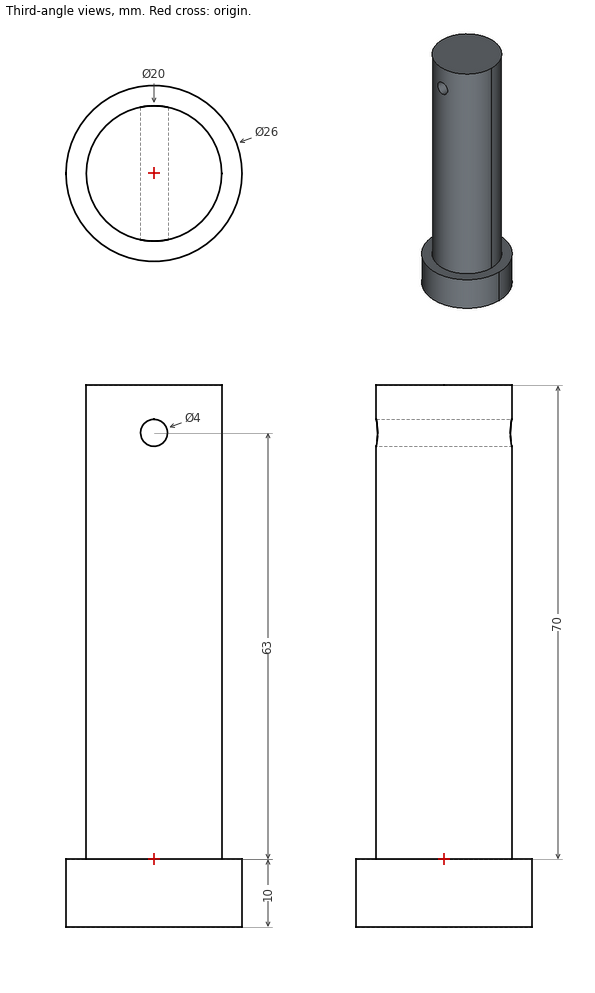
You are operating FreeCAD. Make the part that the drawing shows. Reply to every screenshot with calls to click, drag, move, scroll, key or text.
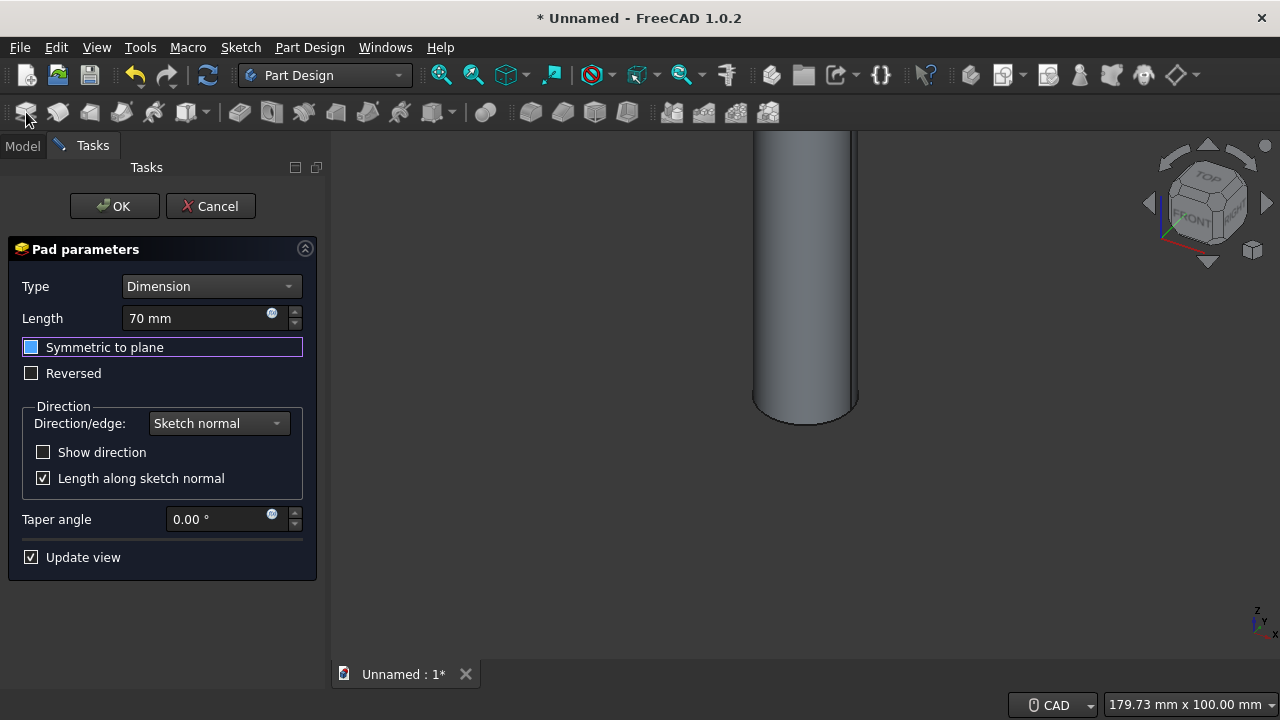
click(115, 206)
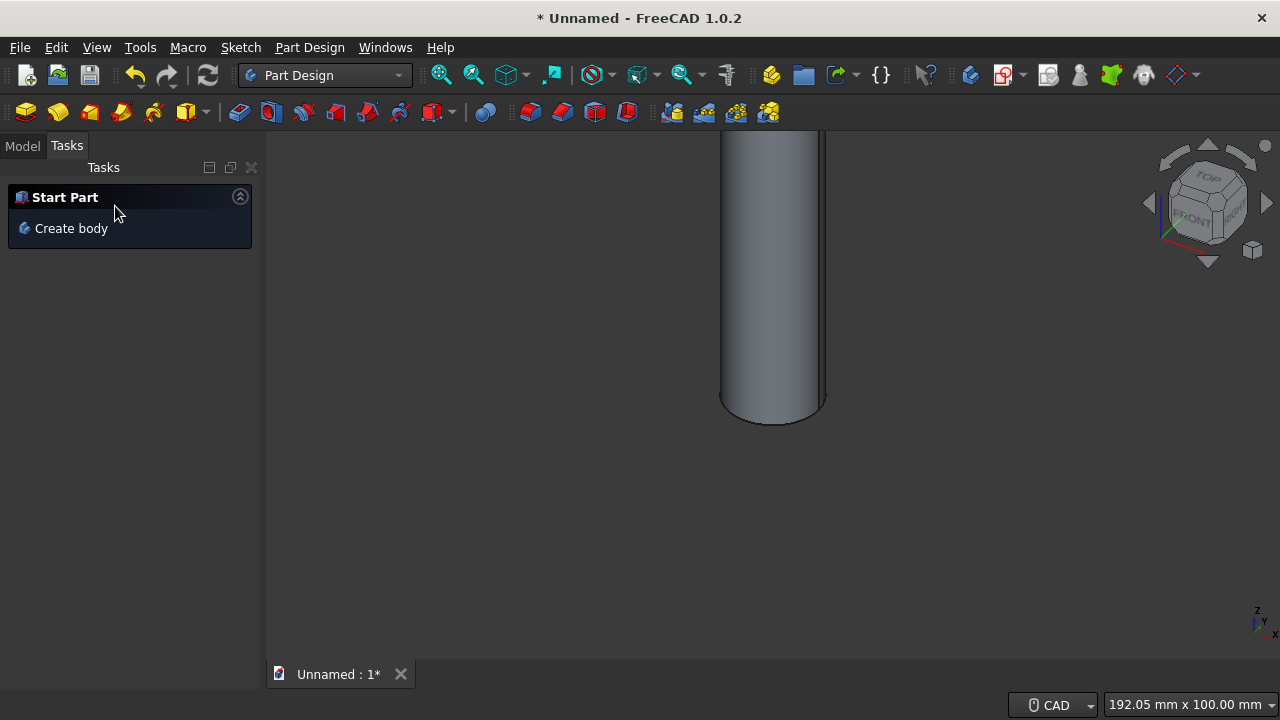
click(442, 76)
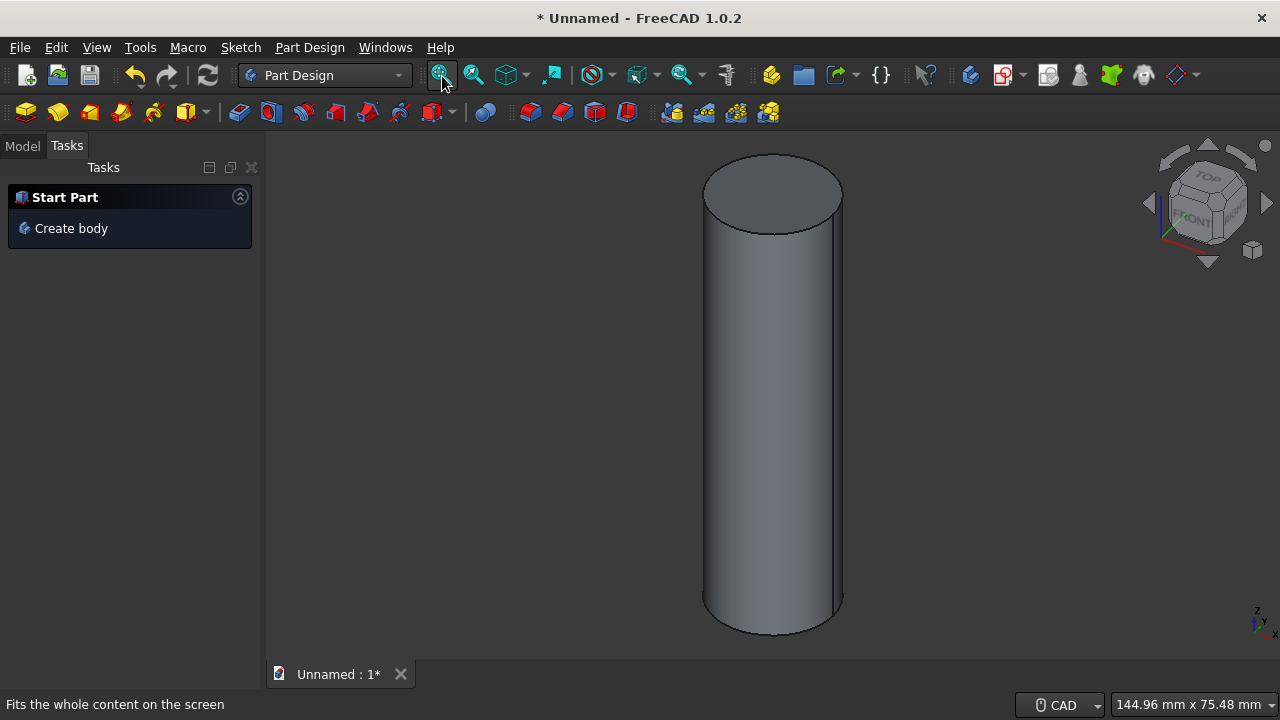
click(1004, 76)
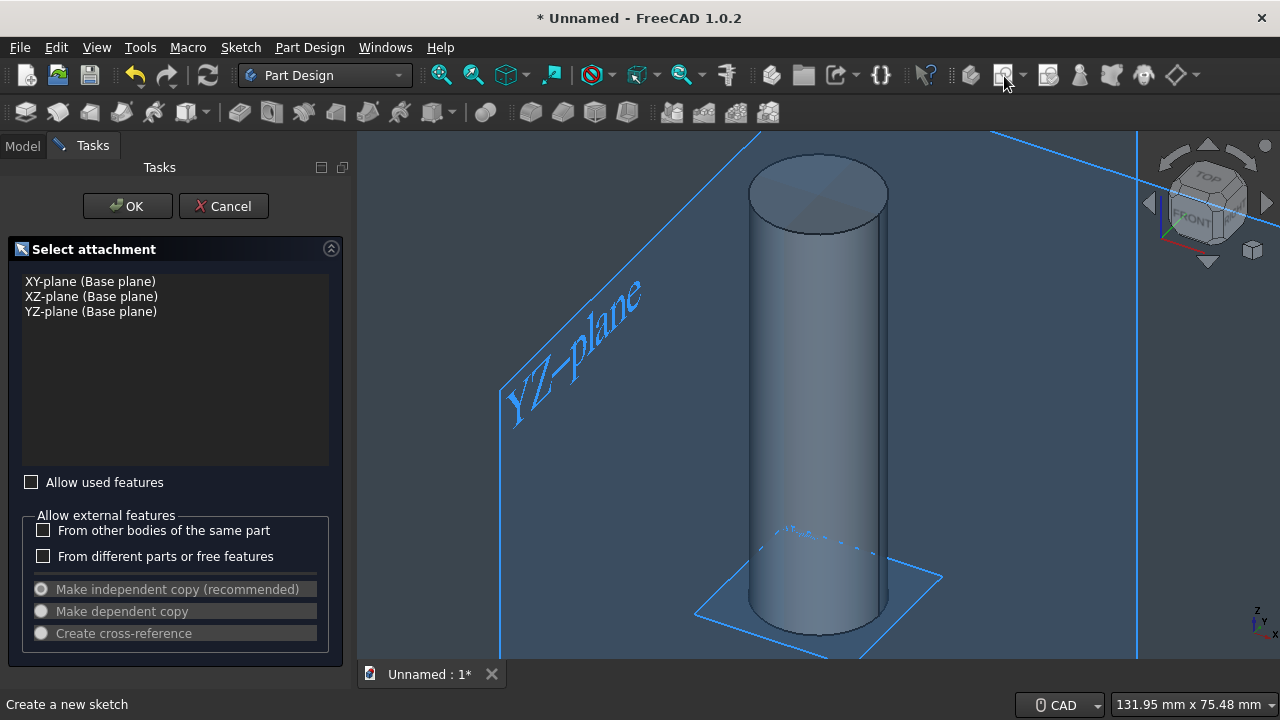
click(82, 282)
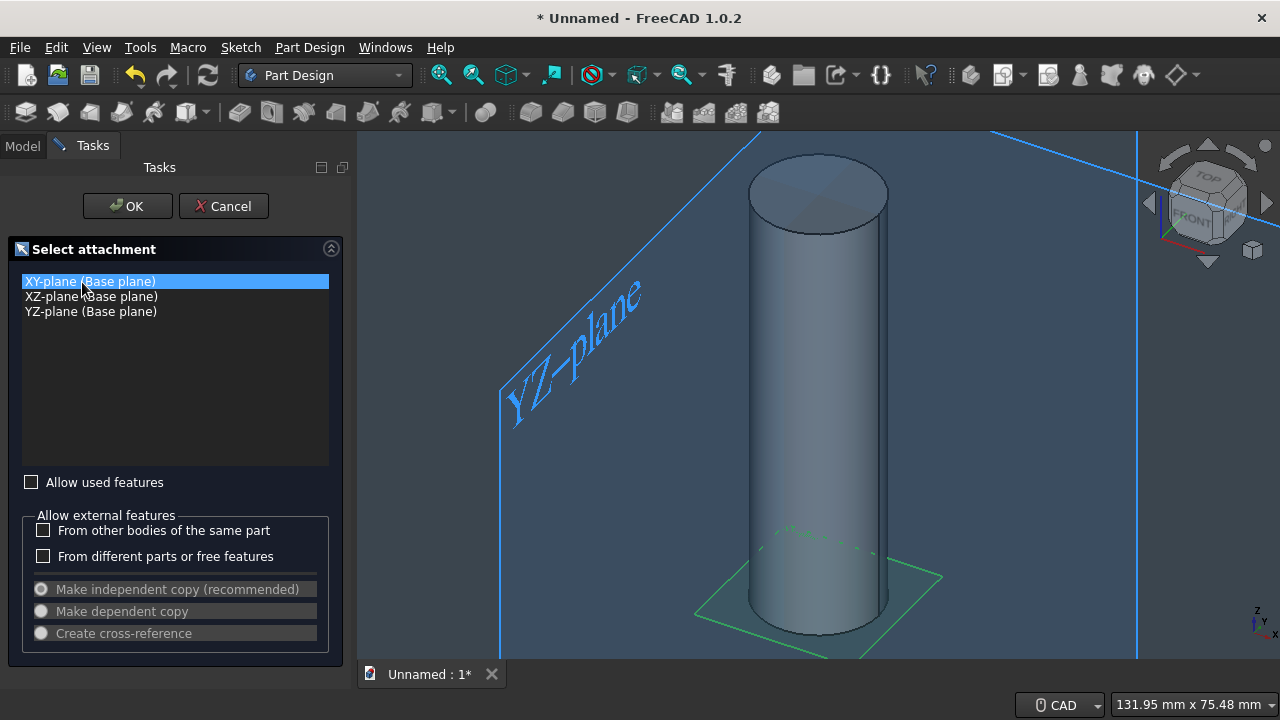
click(128, 206)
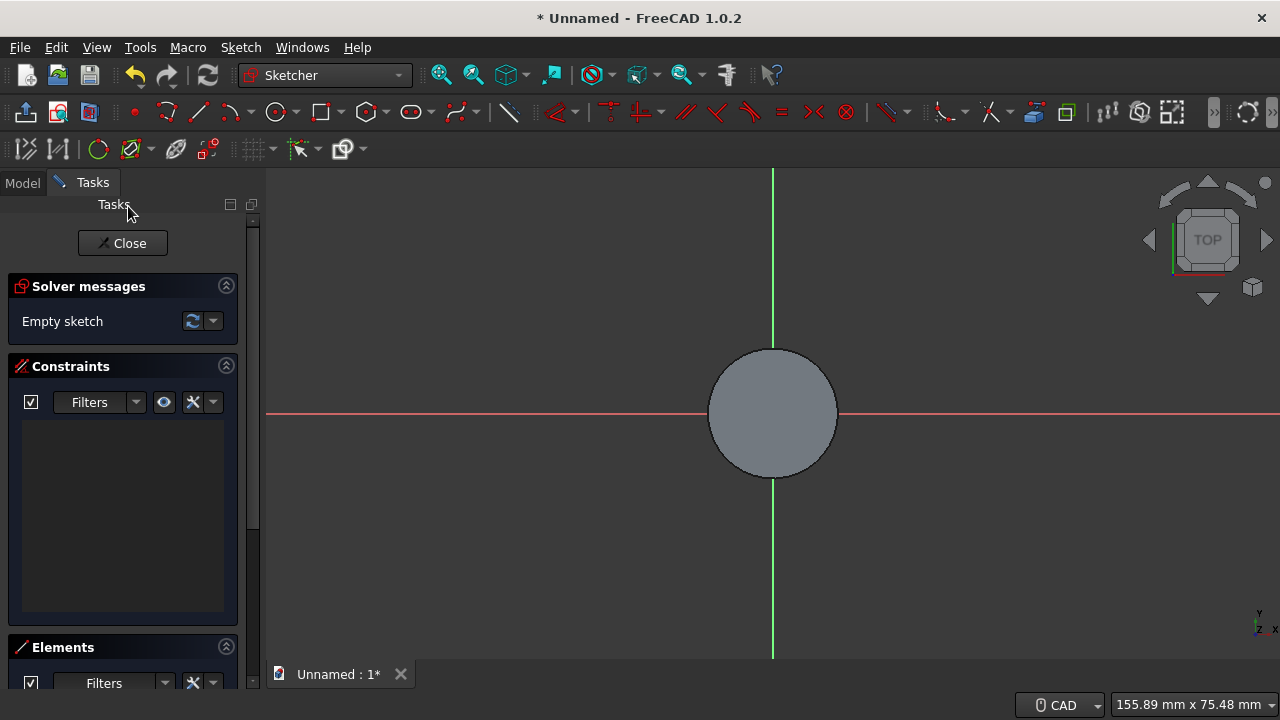
click(90, 112)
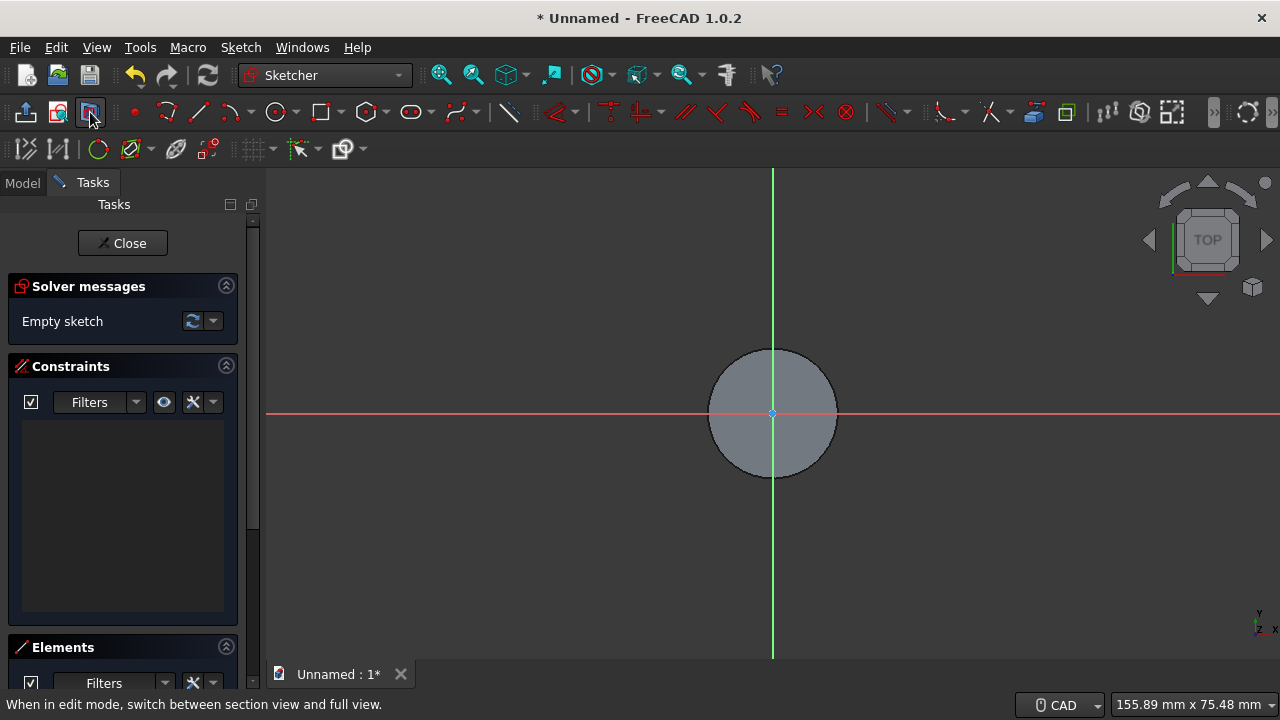
scroll(856, 414, up, 3)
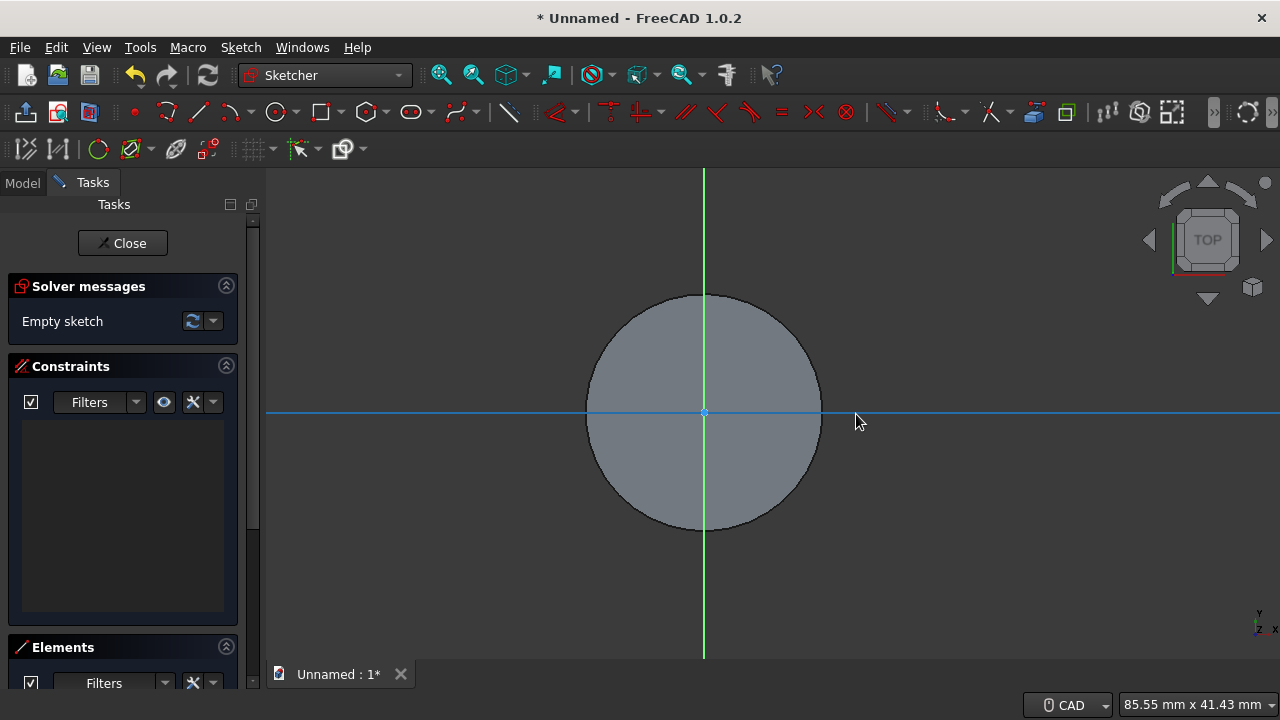
click(276, 112)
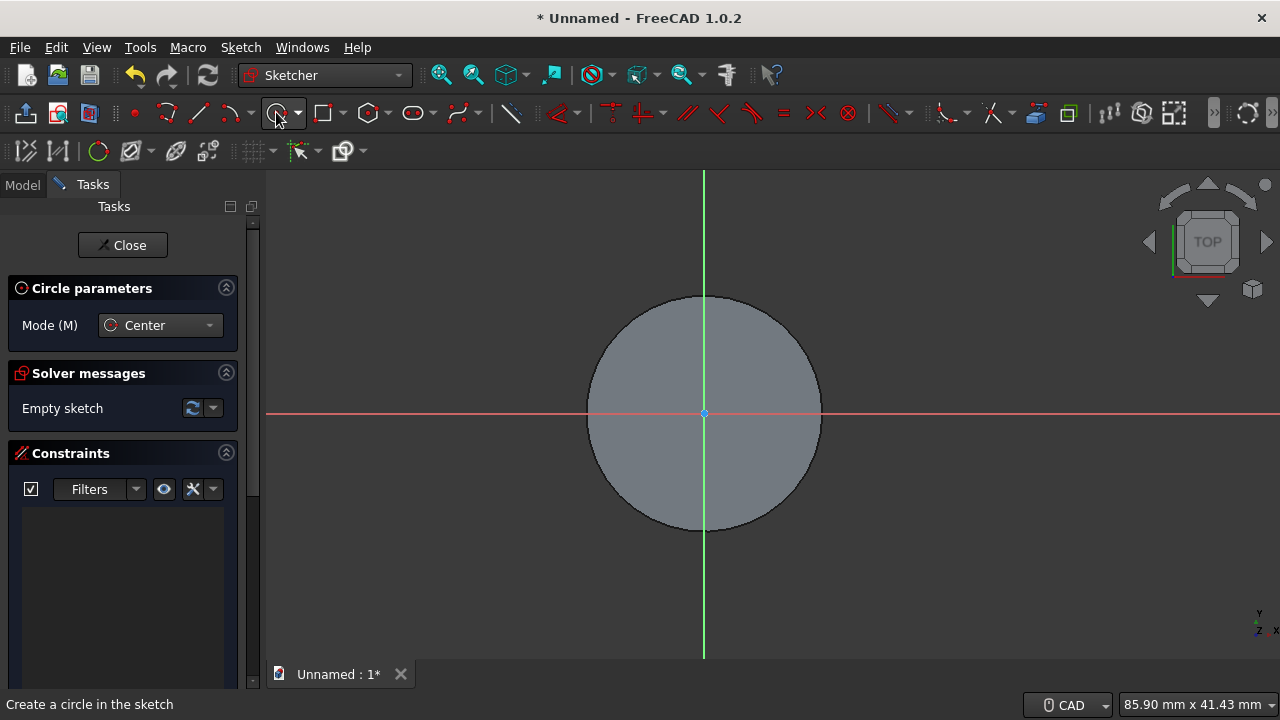
click(704, 414)
move(813, 305)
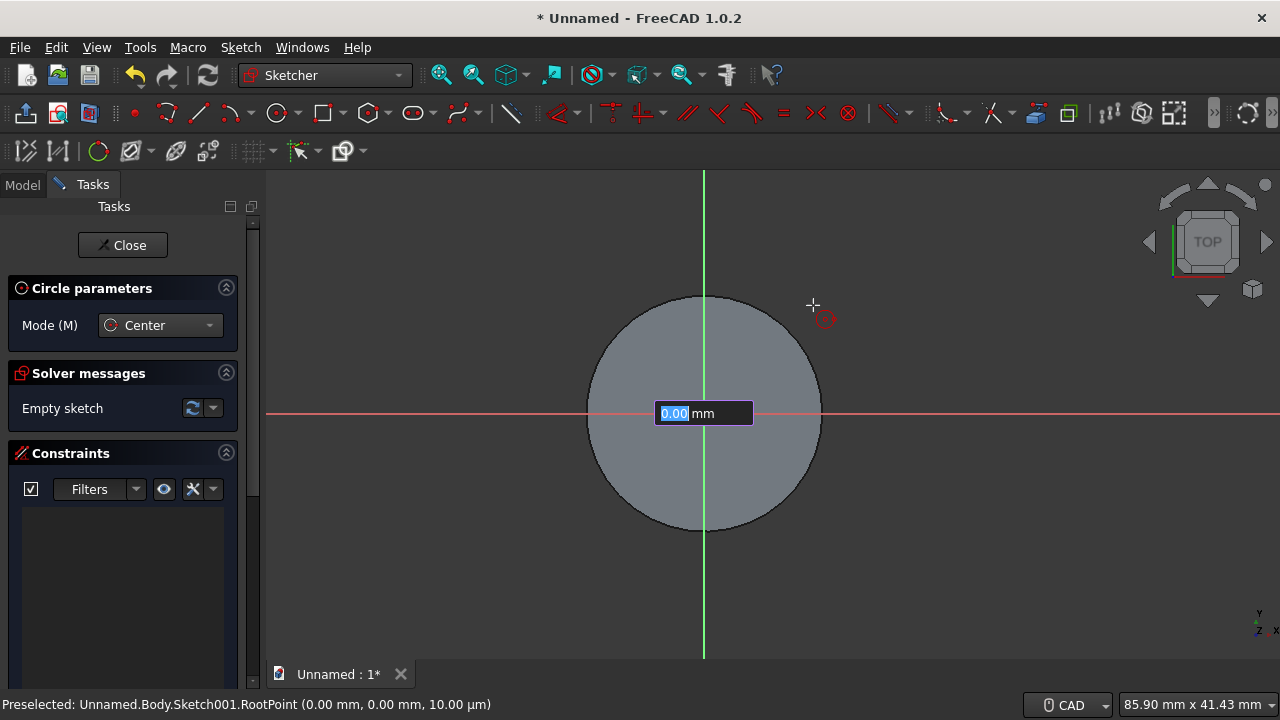
text(26)
key(Return)
key(Escape)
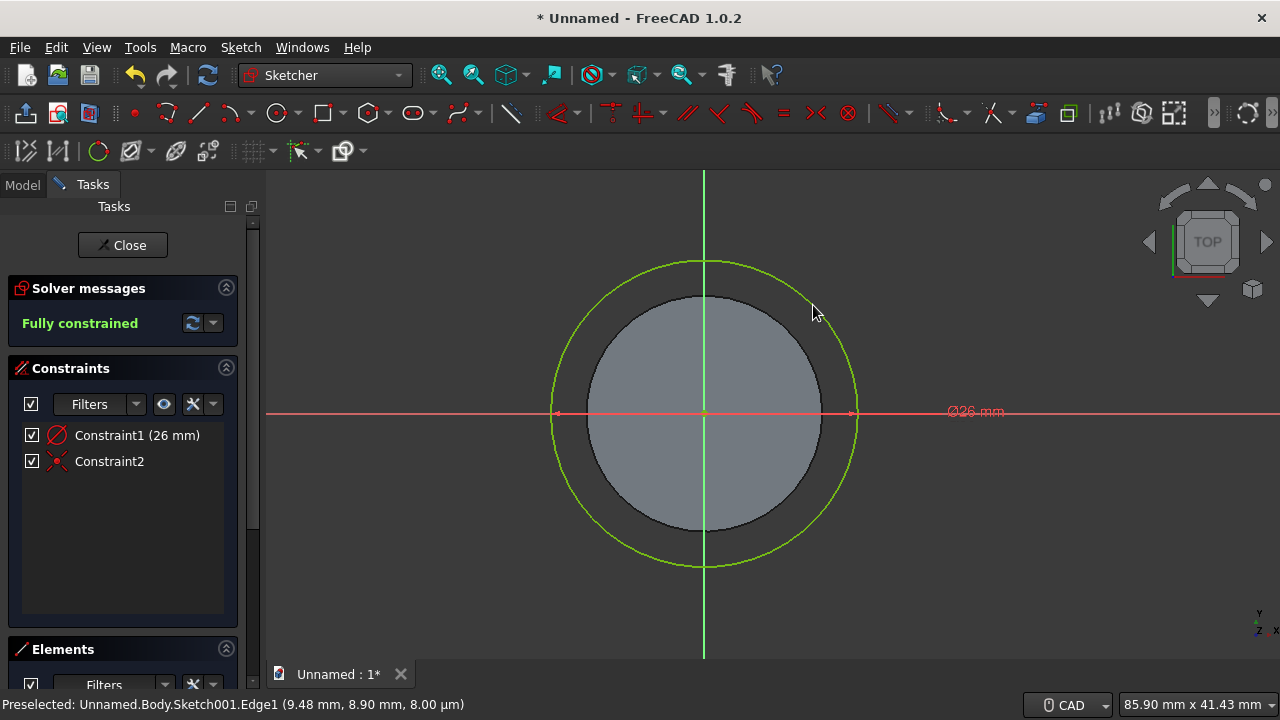
click(123, 245)